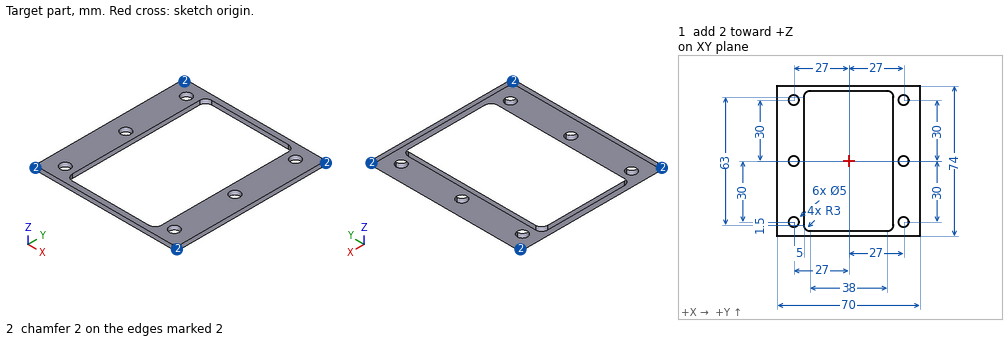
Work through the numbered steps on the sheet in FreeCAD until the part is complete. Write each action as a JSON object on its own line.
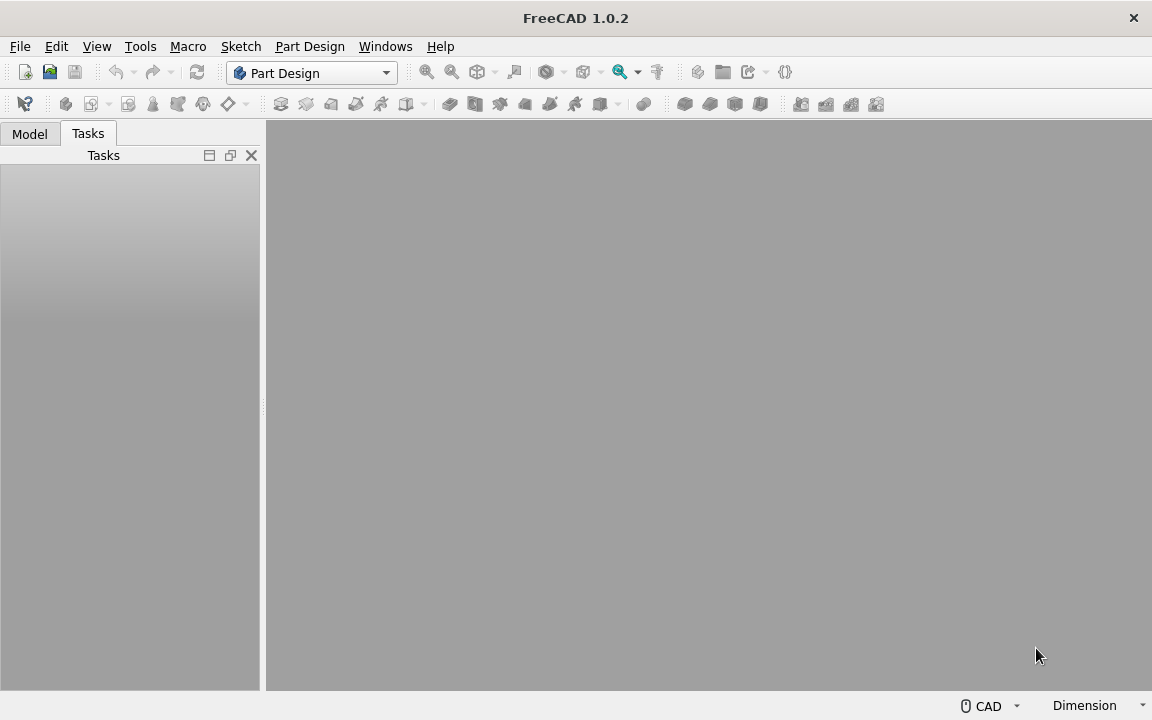
{"action": "left_click", "coordinate": [25, 72]}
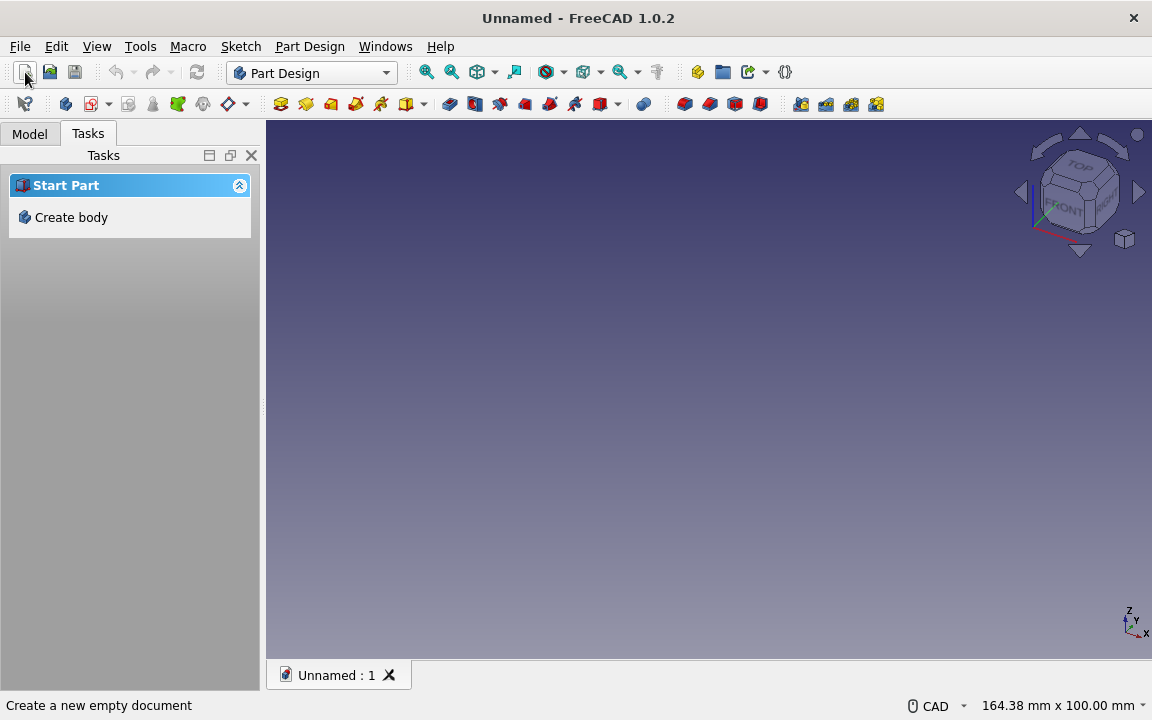
{"action": "left_click", "coordinate": [90, 104]}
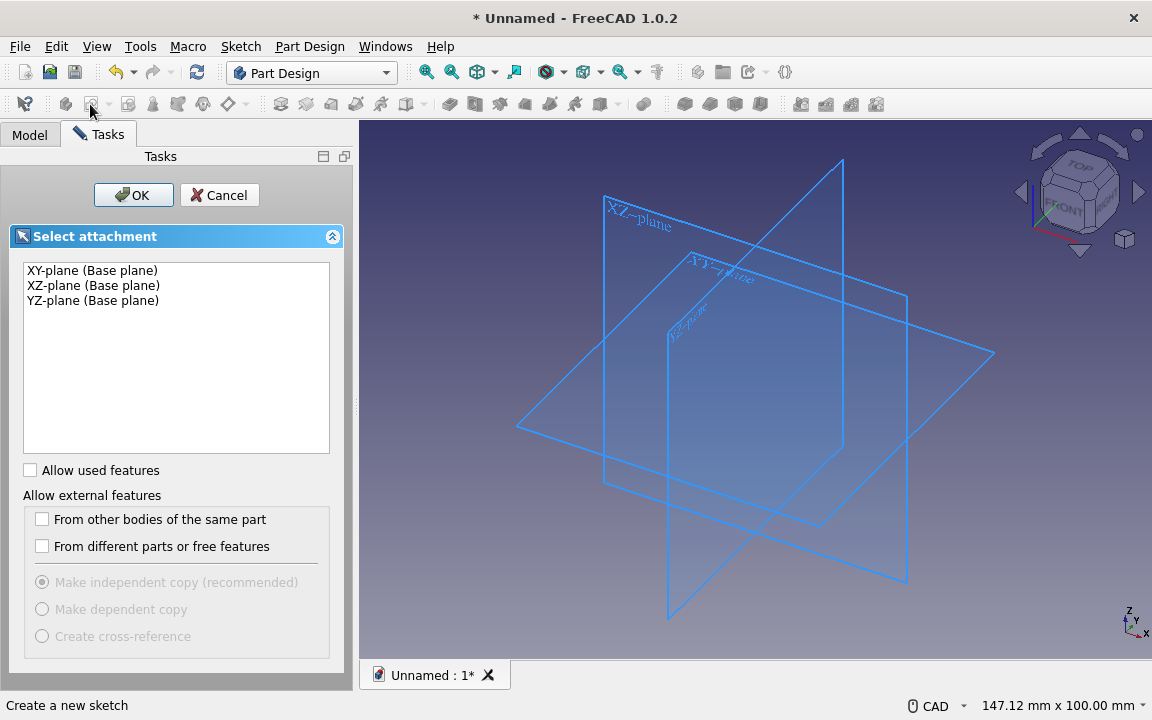
{"action": "left_click", "coordinate": [84, 270]}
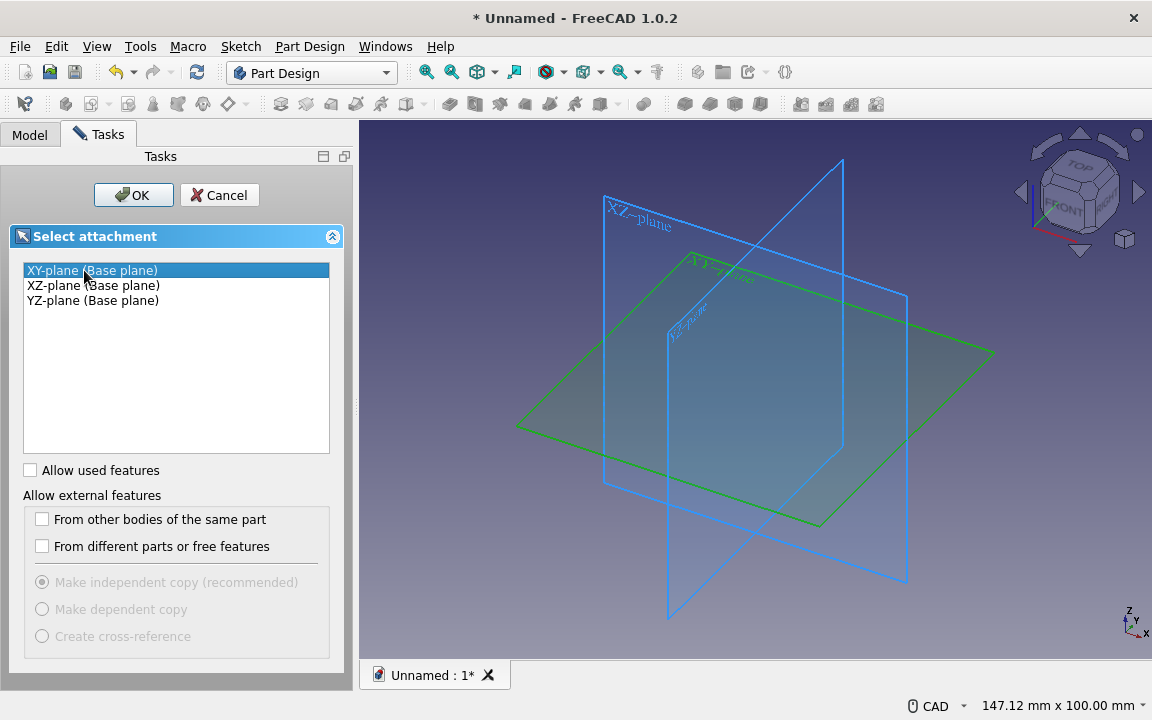
{"action": "left_click", "coordinate": [134, 195]}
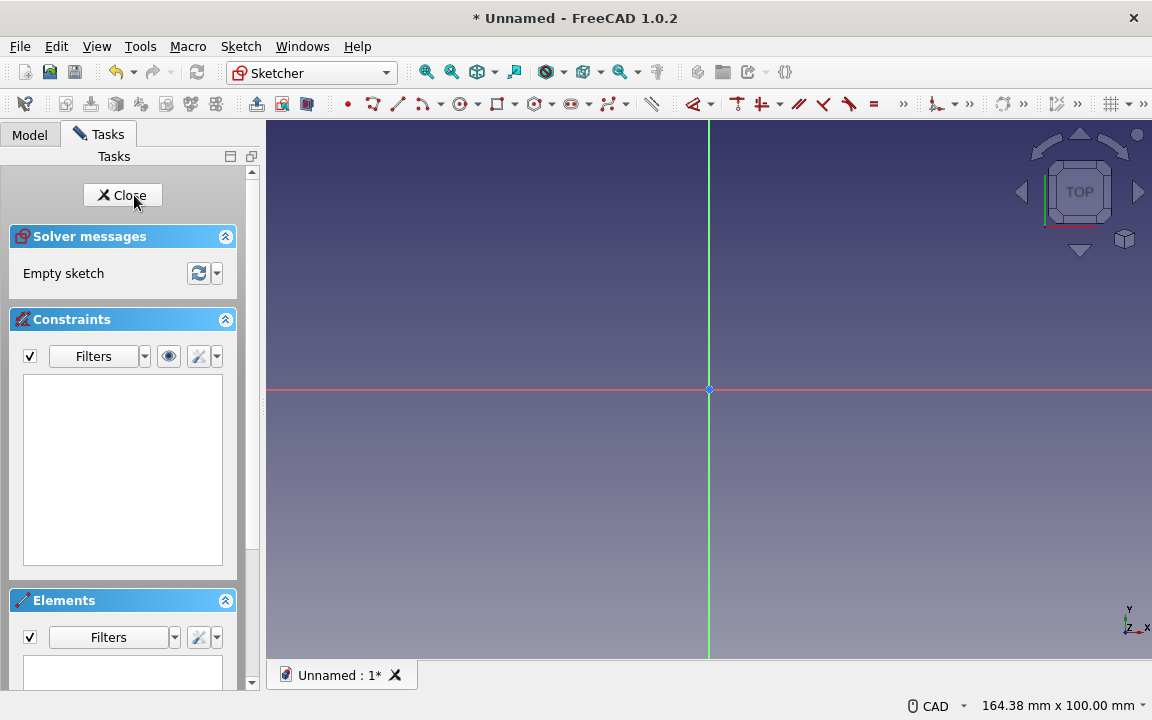
{"action": "key", "text": "g v"}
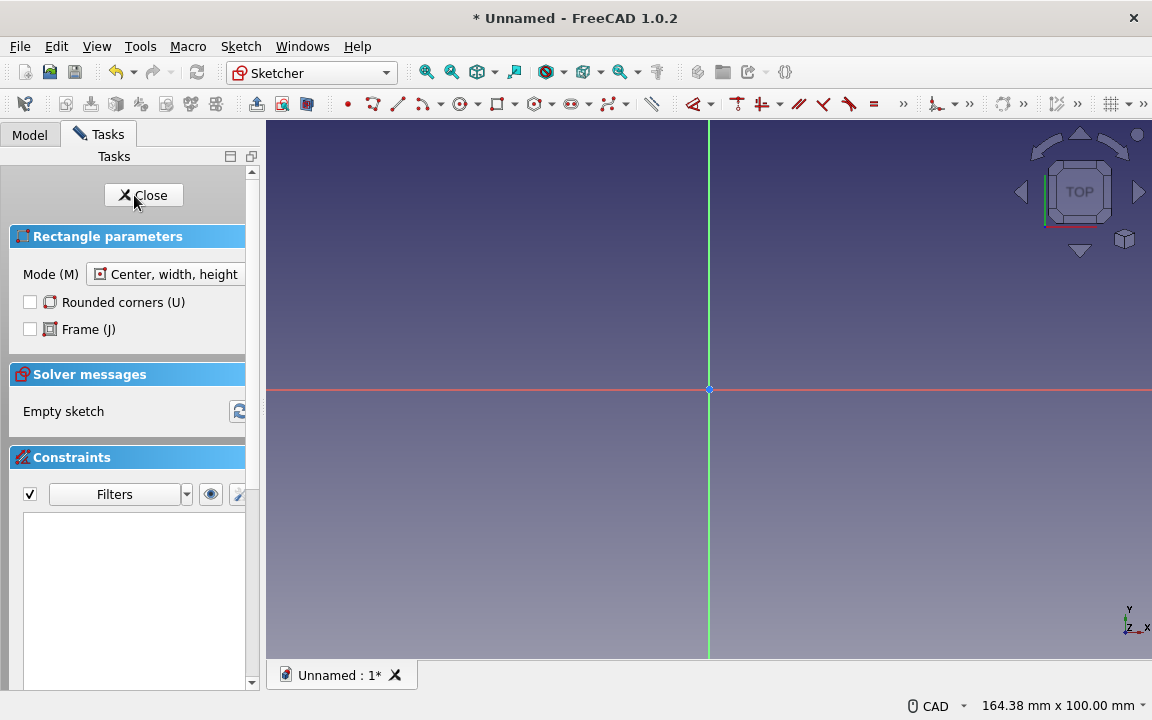
{"action": "left_click", "coordinate": [709, 390]}
{"action": "mouse_move", "coordinate": [898, 190]}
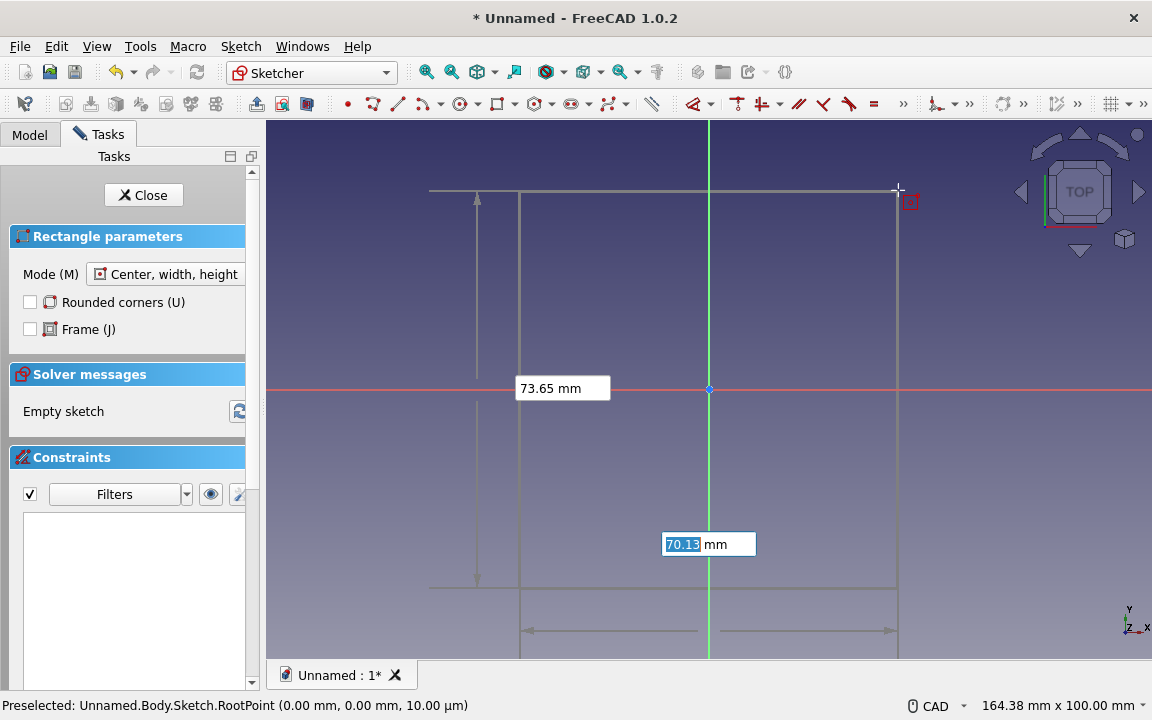
{"action": "type", "text": "70"}
{"action": "key", "text": "Tab"}
{"action": "type", "text": "74"}
{"action": "key", "text": "Return"}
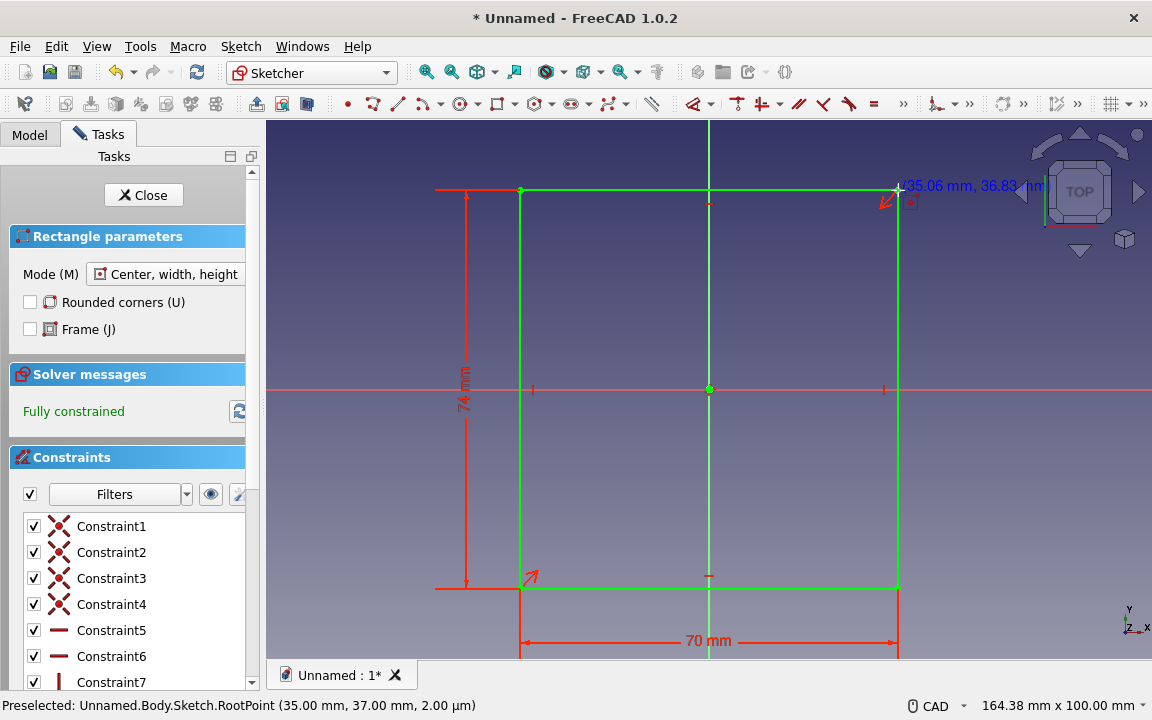
{"action": "left_click", "coordinate": [398, 104]}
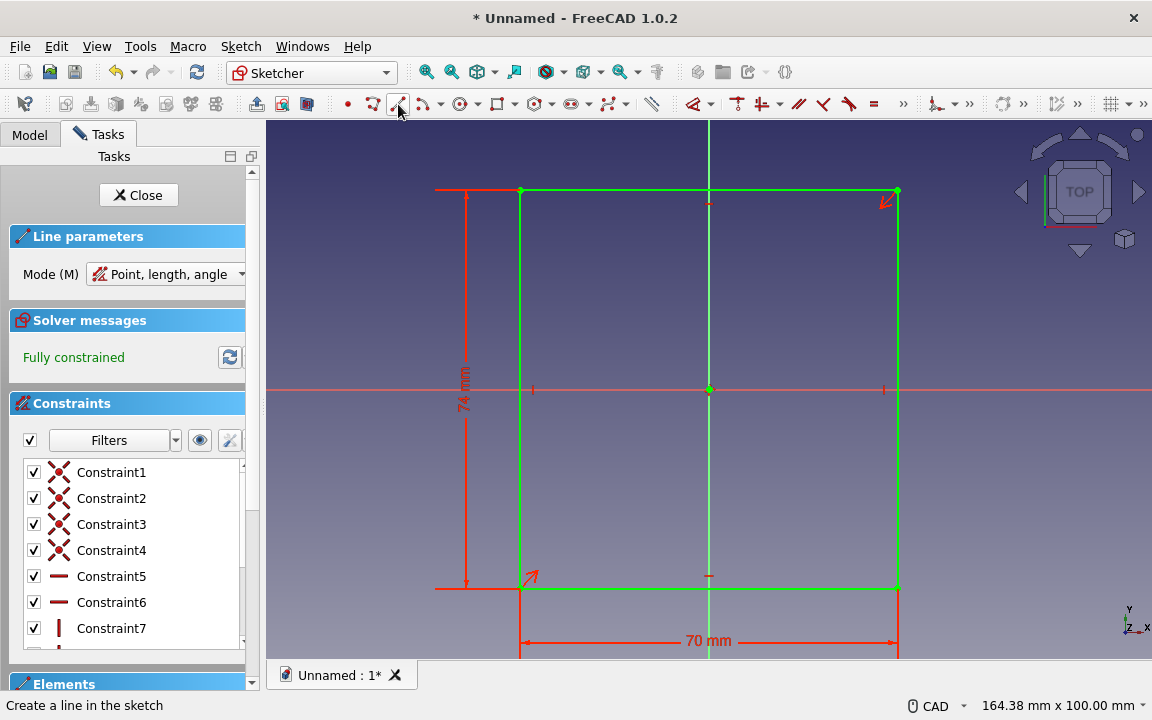
{"action": "left_click", "coordinate": [811, 575]}
{"action": "left_click", "coordinate": [607, 575]}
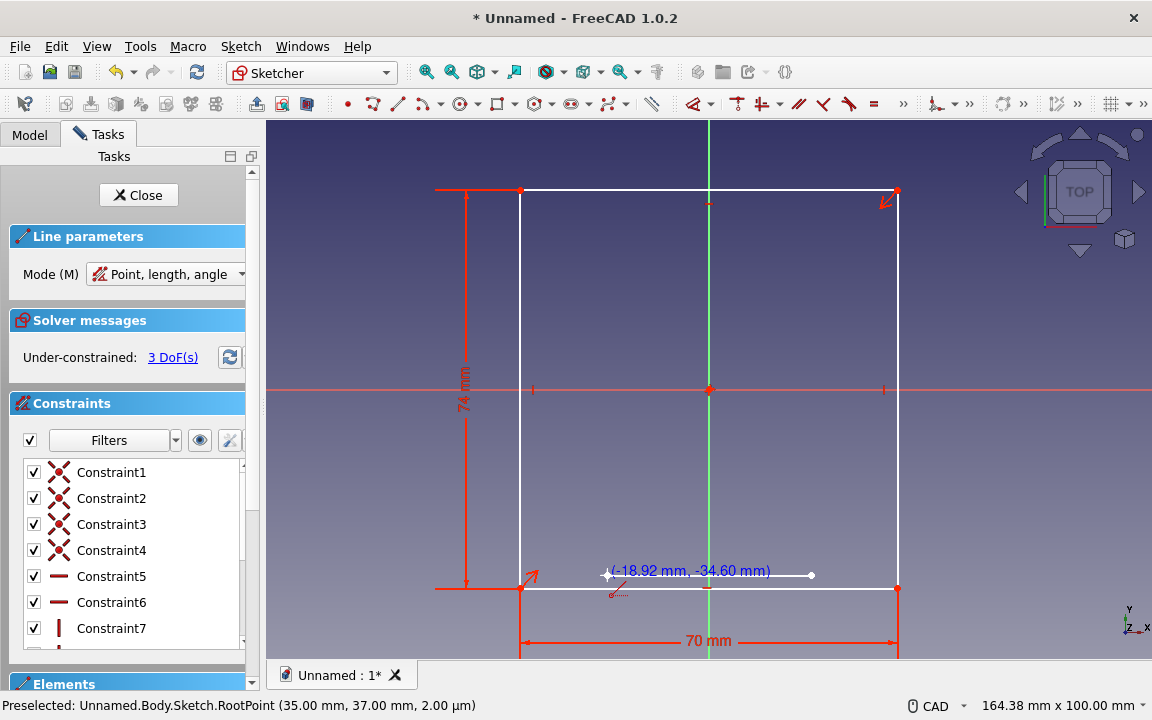
{"action": "left_click", "coordinate": [590, 559]}
{"action": "left_click", "coordinate": [590, 220]}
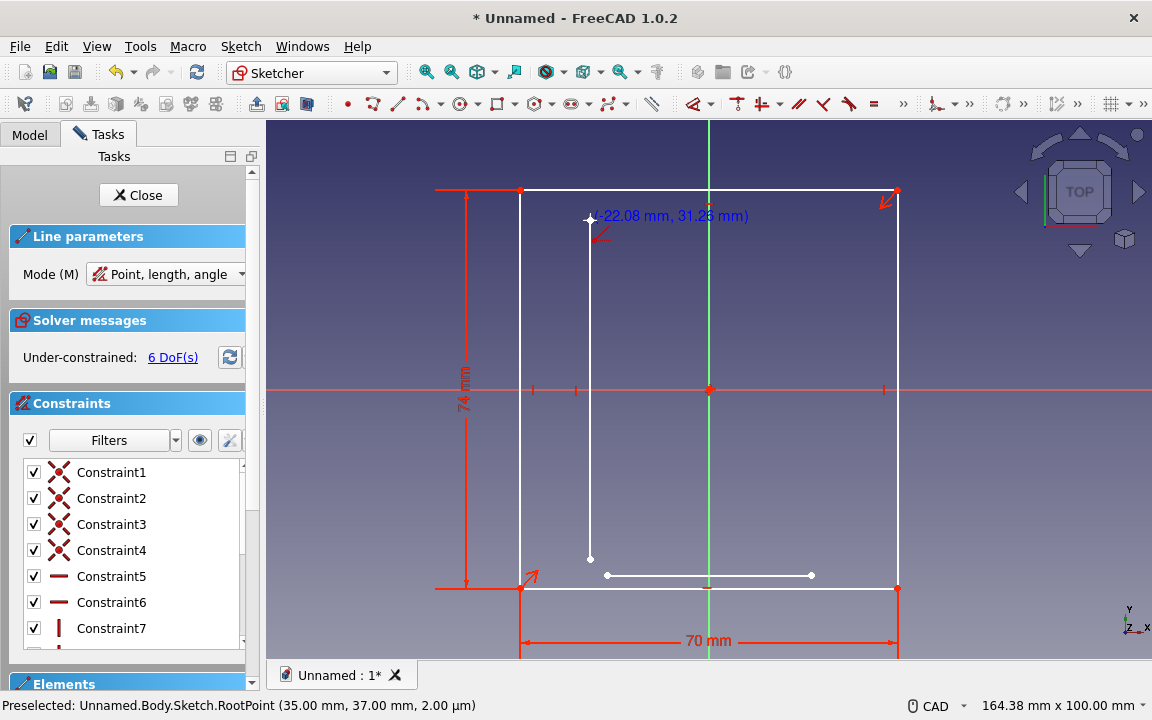
{"action": "left_click", "coordinate": [607, 204]}
{"action": "left_click", "coordinate": [811, 204]}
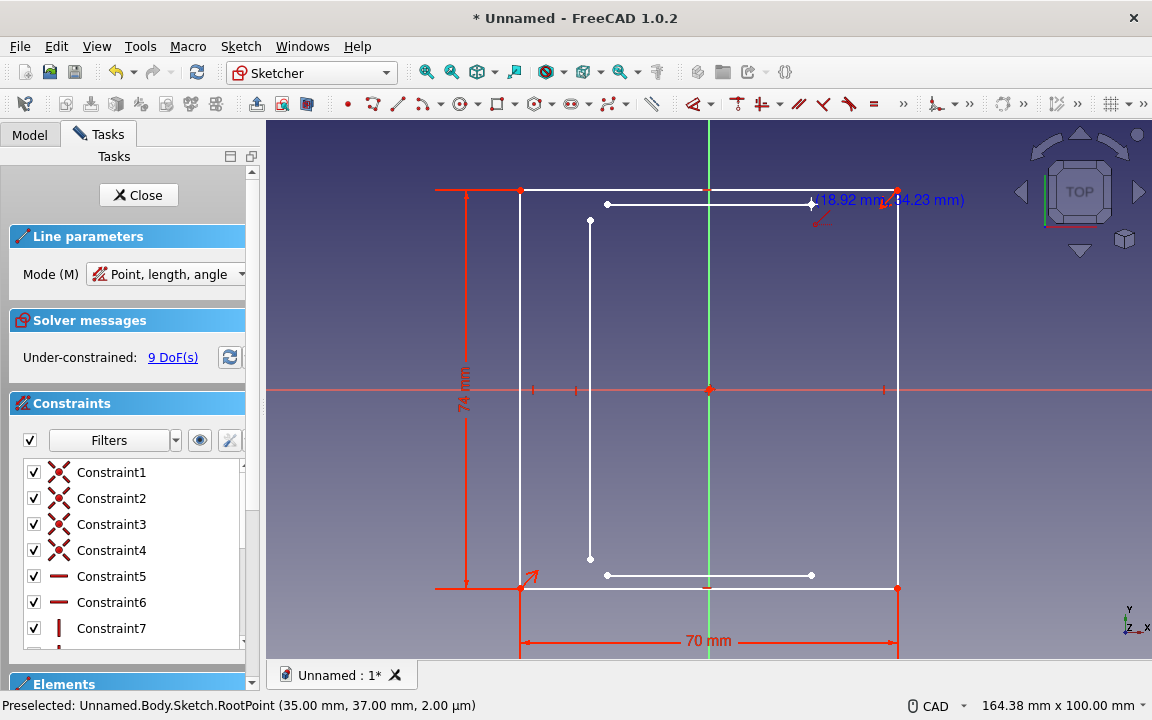
{"action": "left_click", "coordinate": [828, 220]}
{"action": "left_click", "coordinate": [828, 559]}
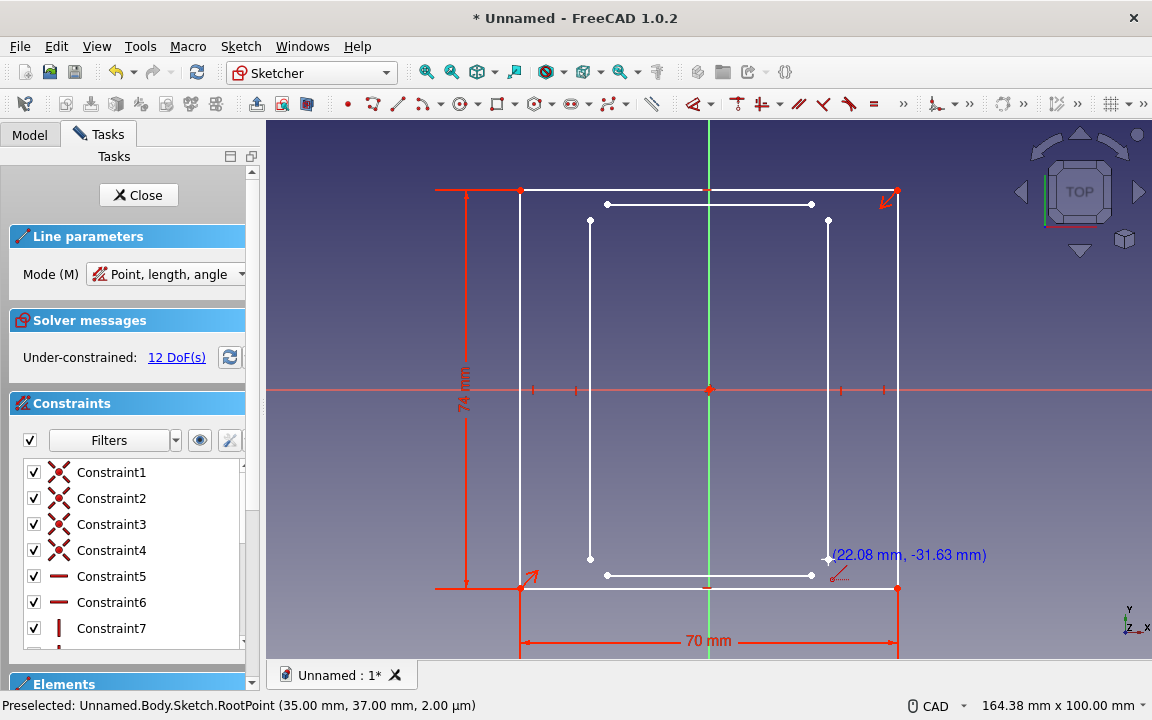
{"action": "left_click", "coordinate": [440, 104]}